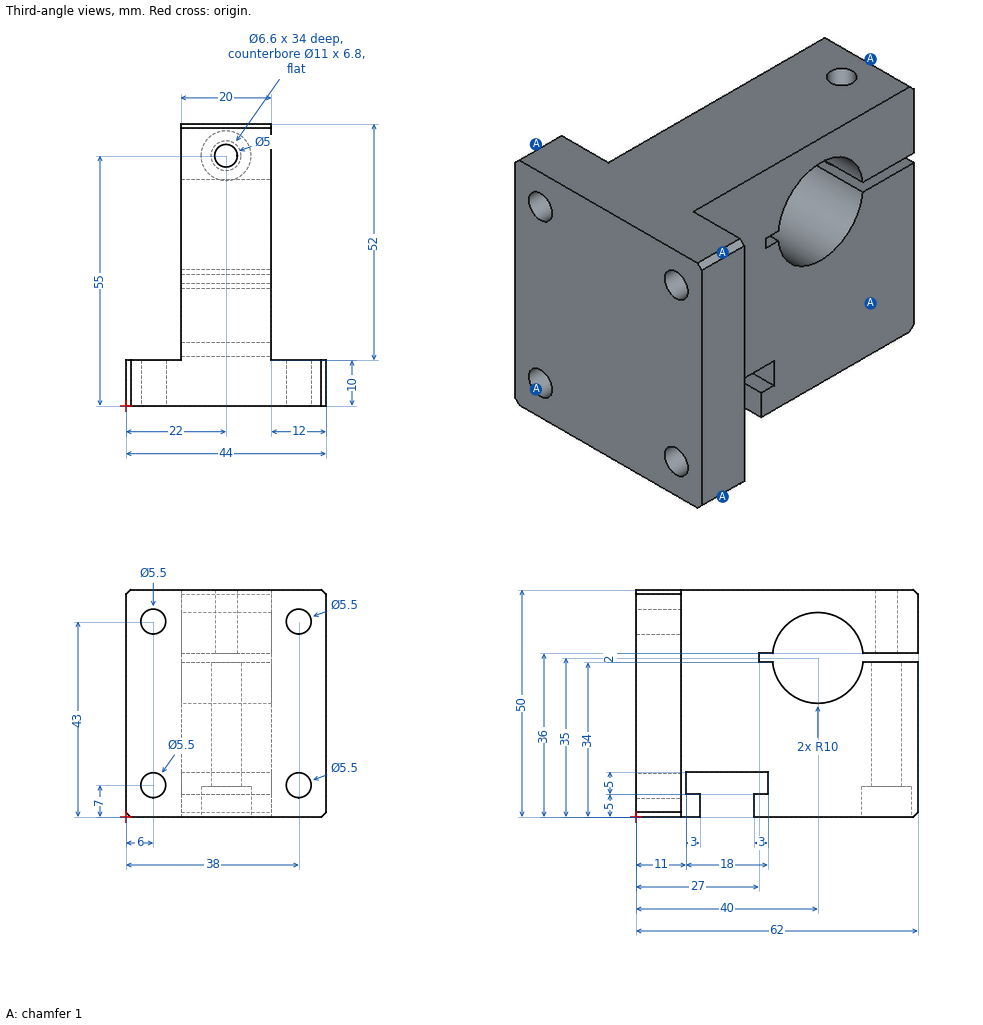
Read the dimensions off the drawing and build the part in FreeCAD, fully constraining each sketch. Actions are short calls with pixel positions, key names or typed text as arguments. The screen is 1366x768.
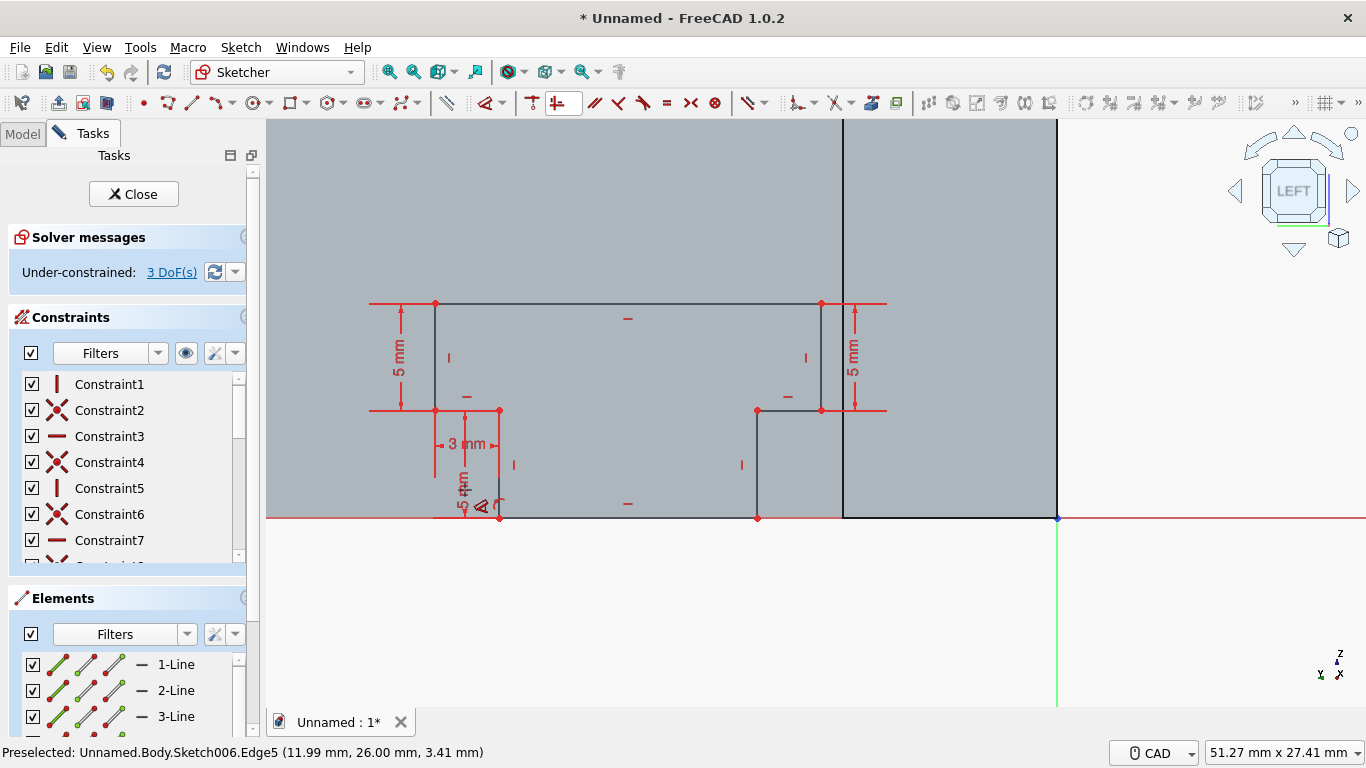
click(776, 411)
click(789, 445)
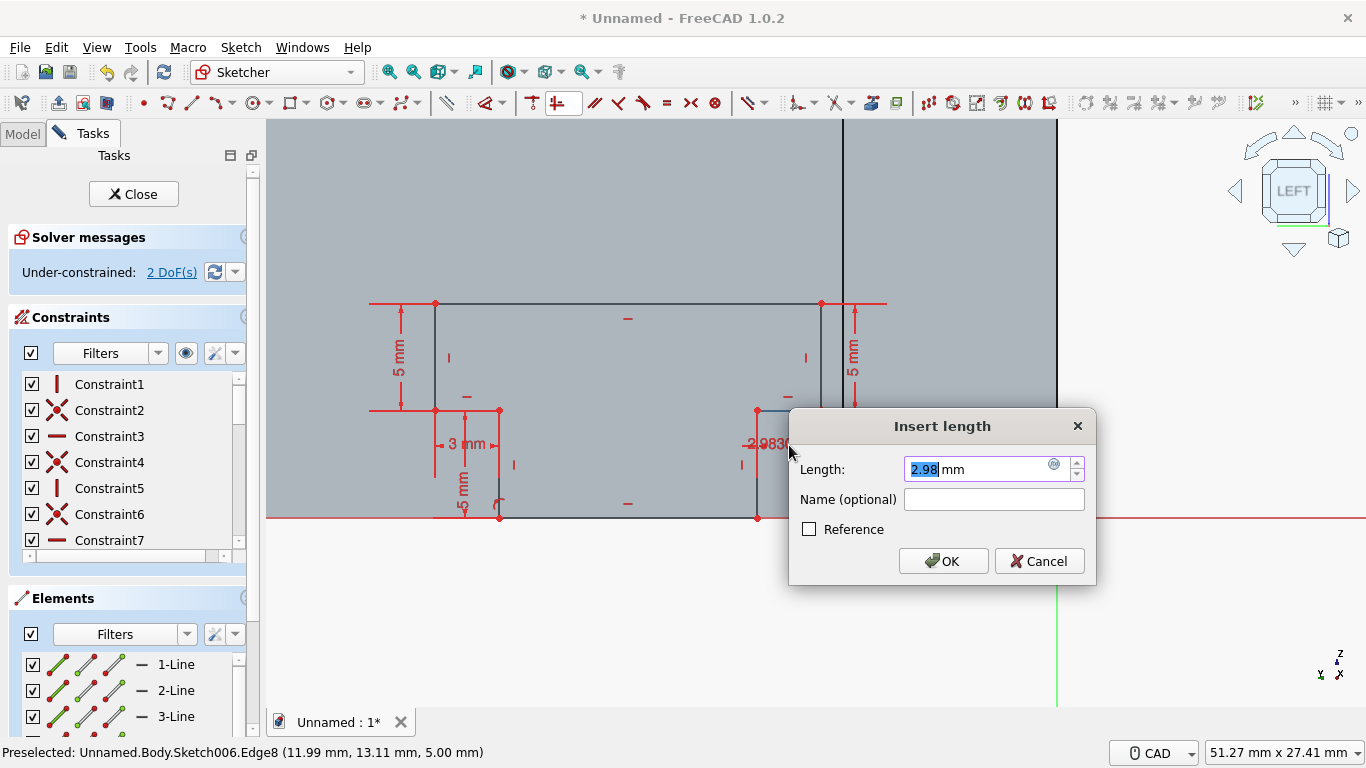
text(3)
key(Return)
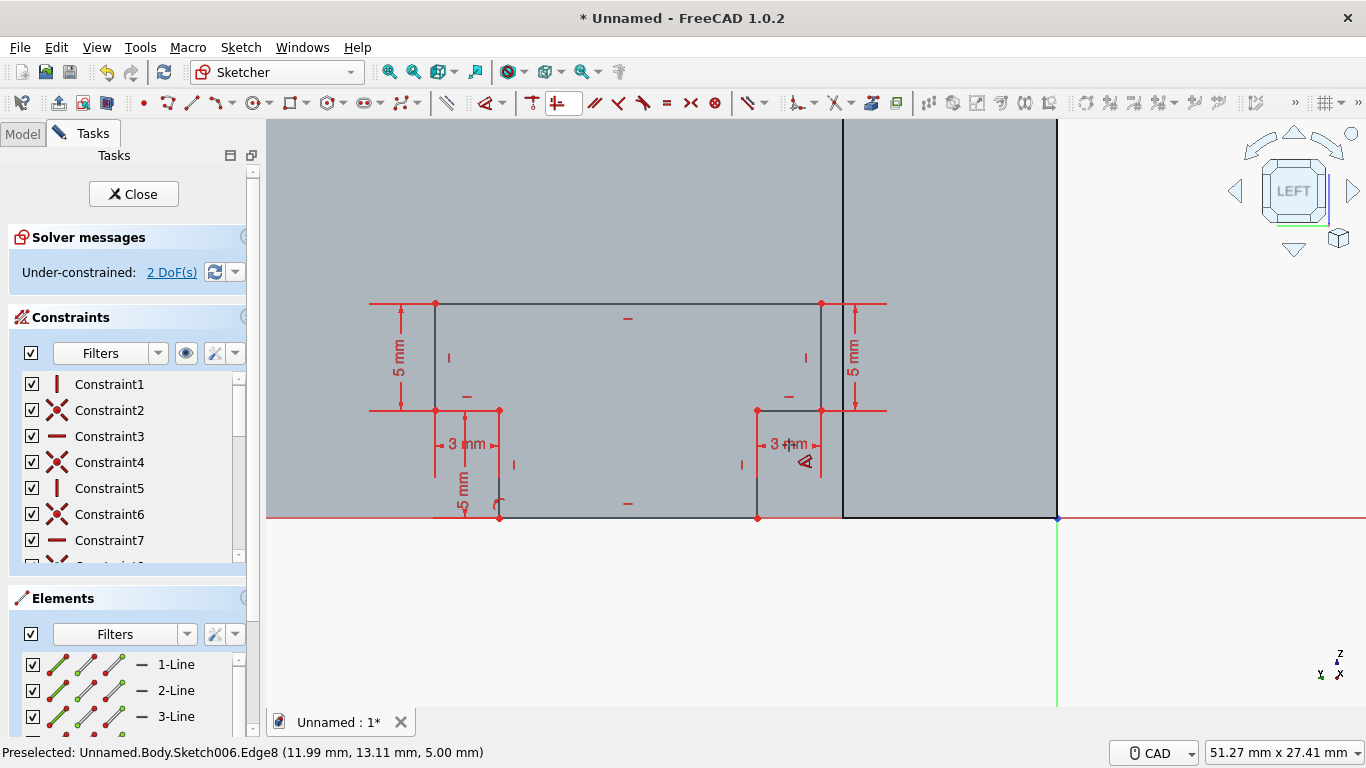
click(705, 304)
click(628, 270)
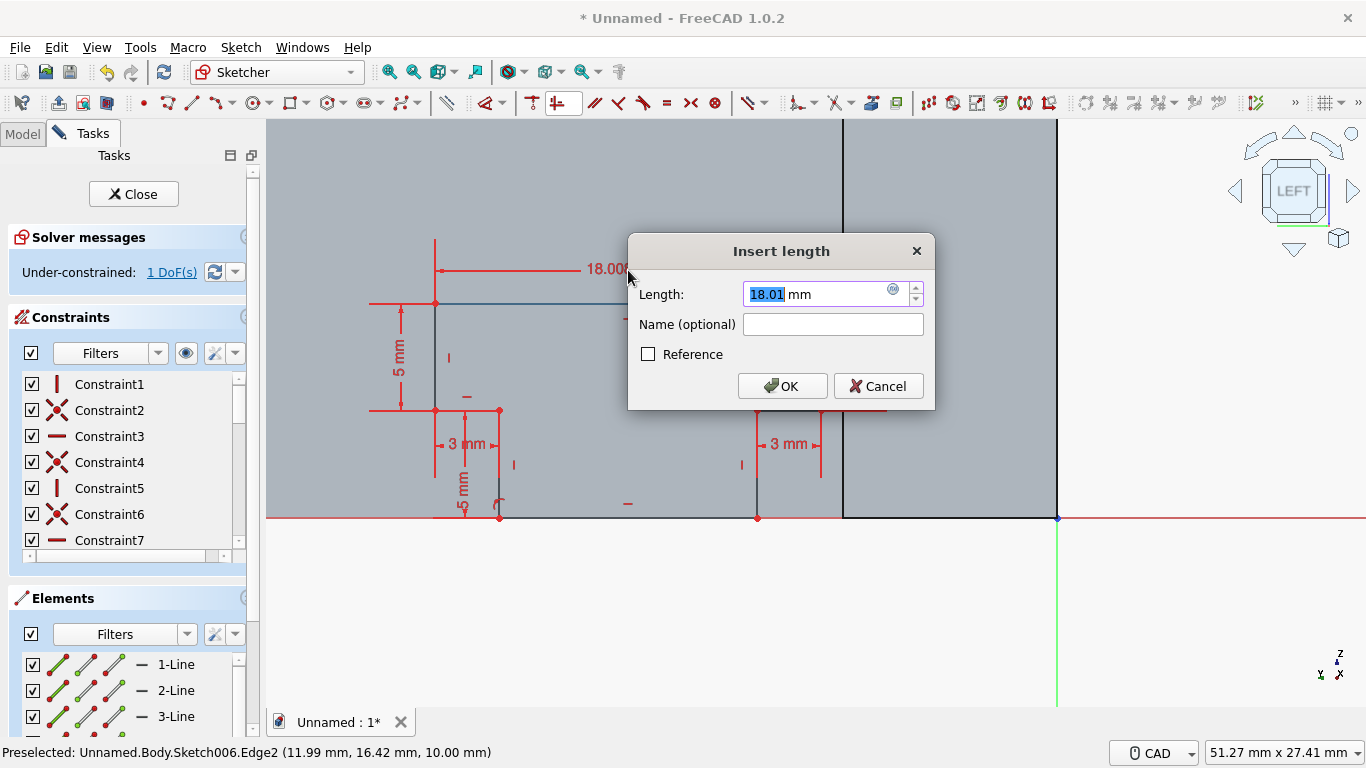
text(18)
key(Return)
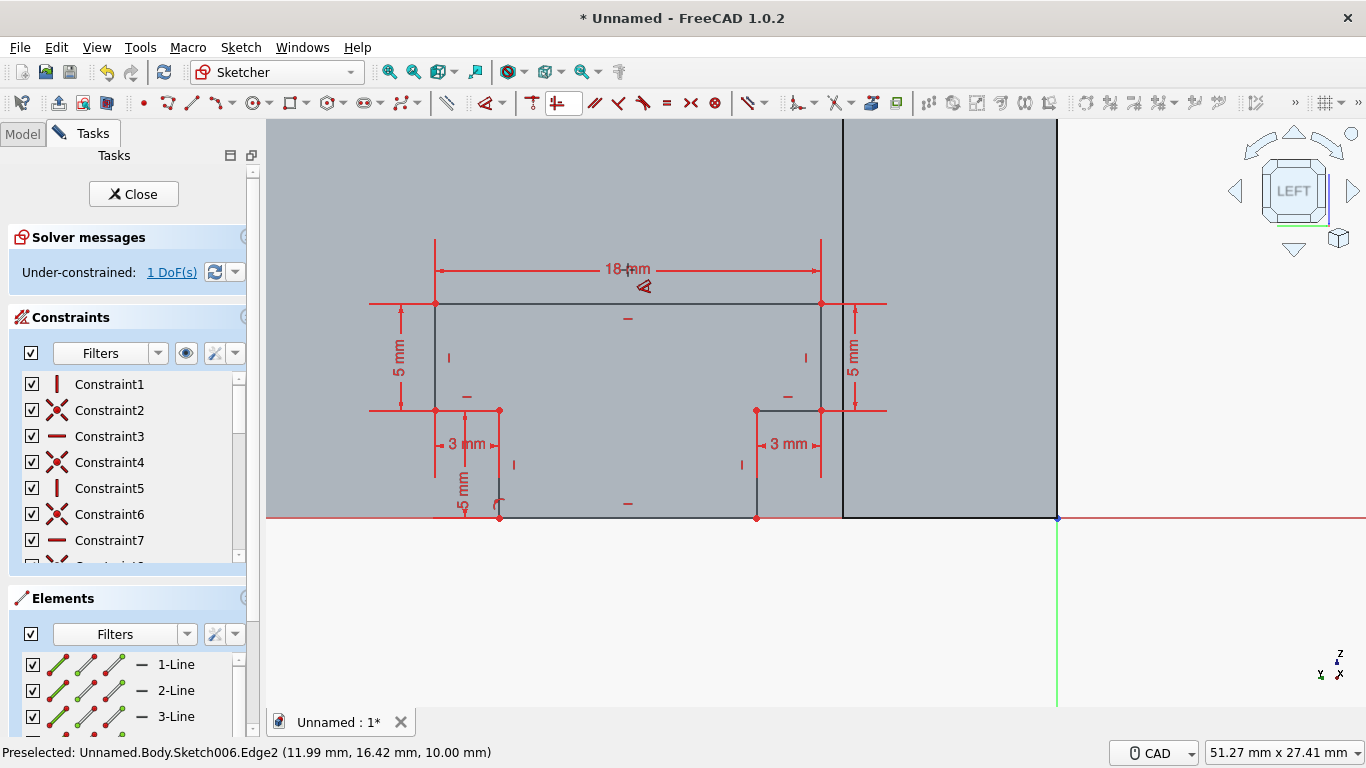
click(821, 411)
click(939, 552)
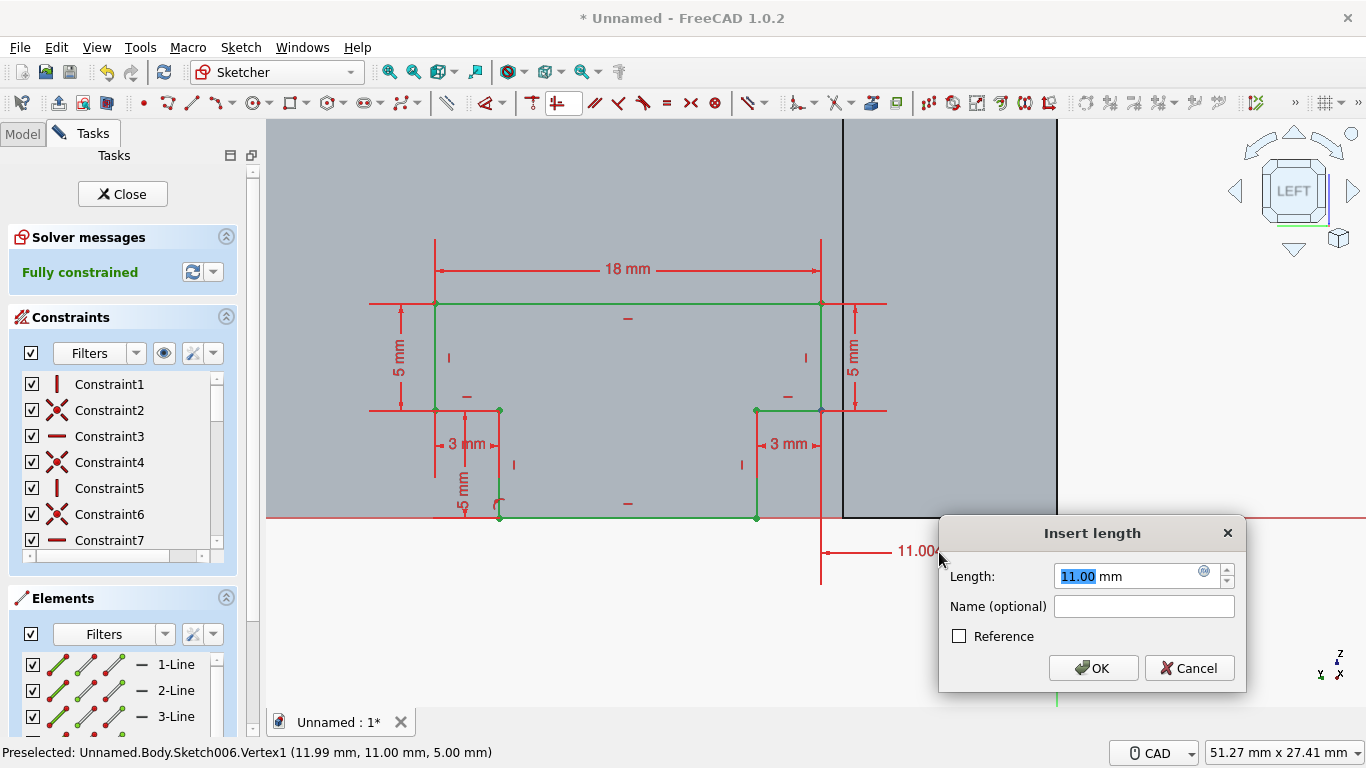
text(11)
key(Return)
key(Escape)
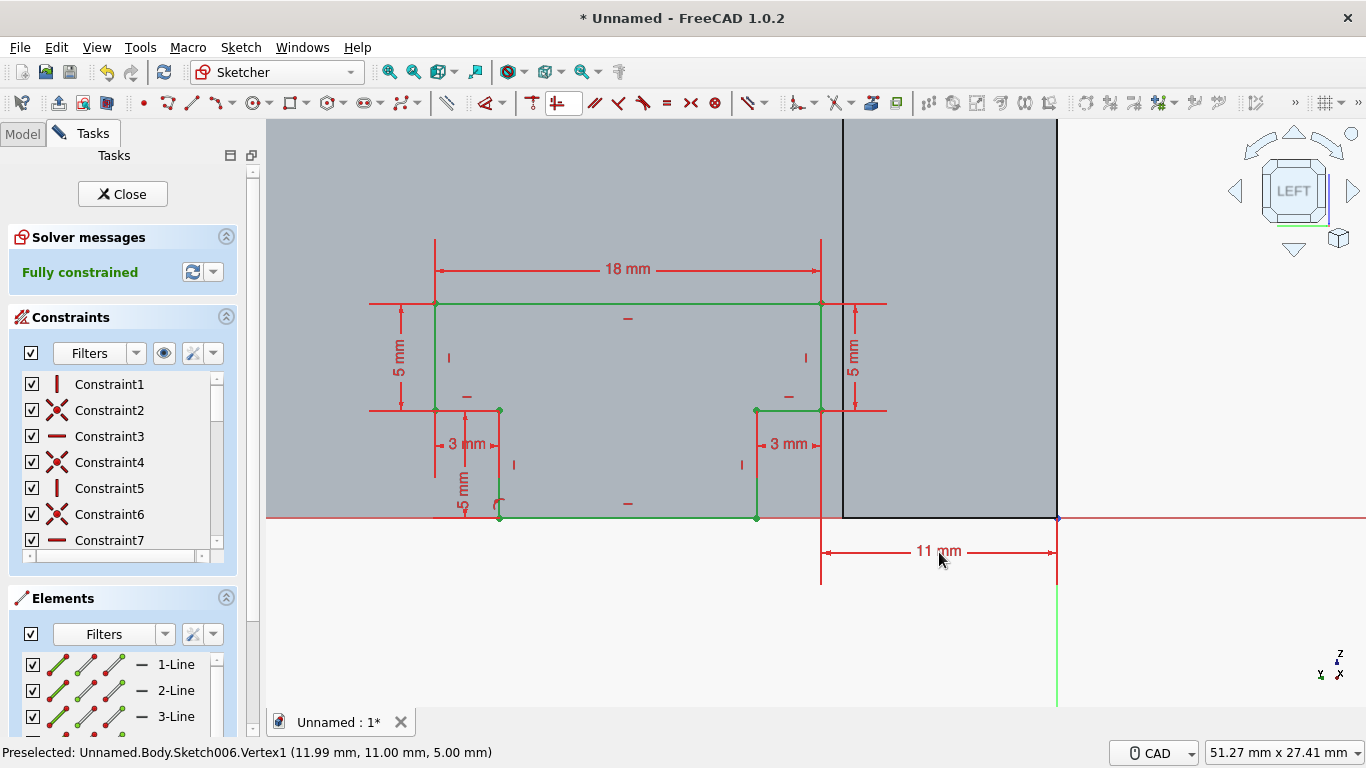
click(123, 194)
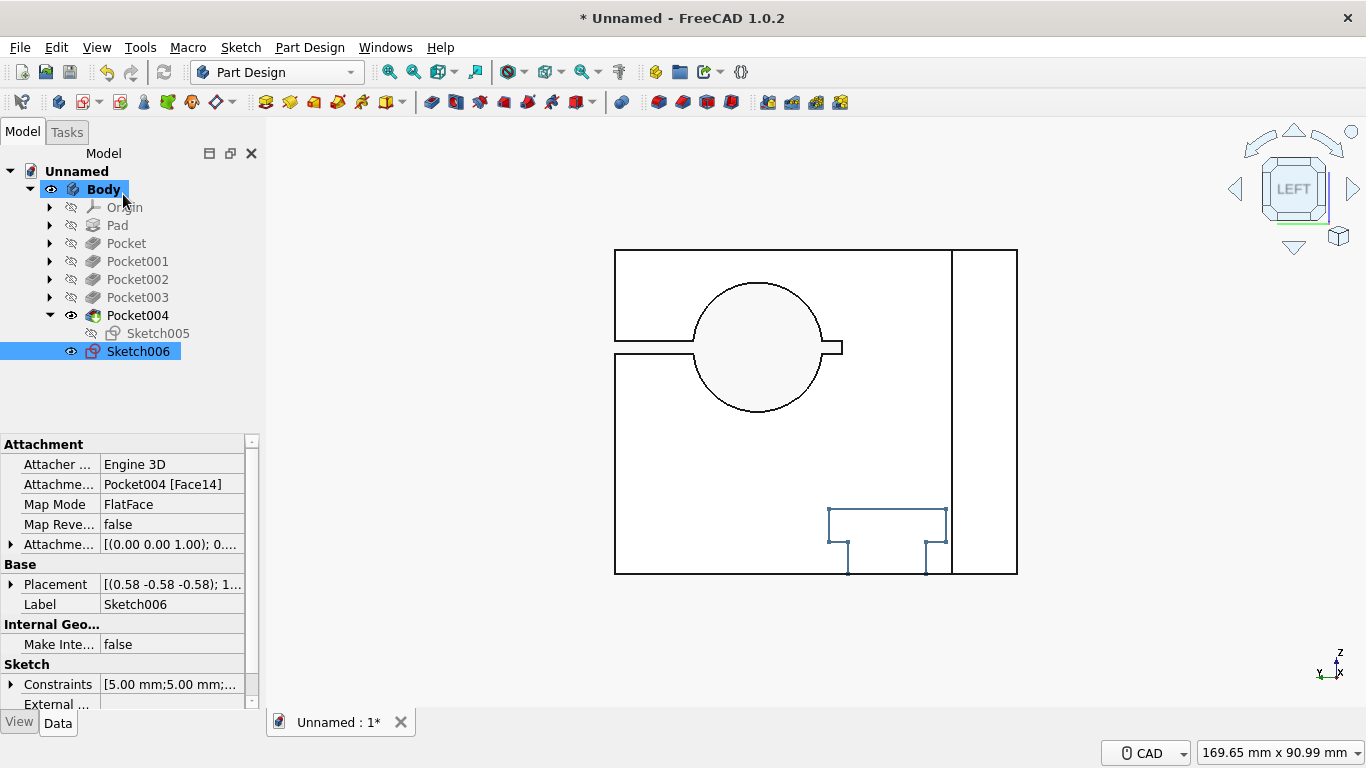
click(432, 102)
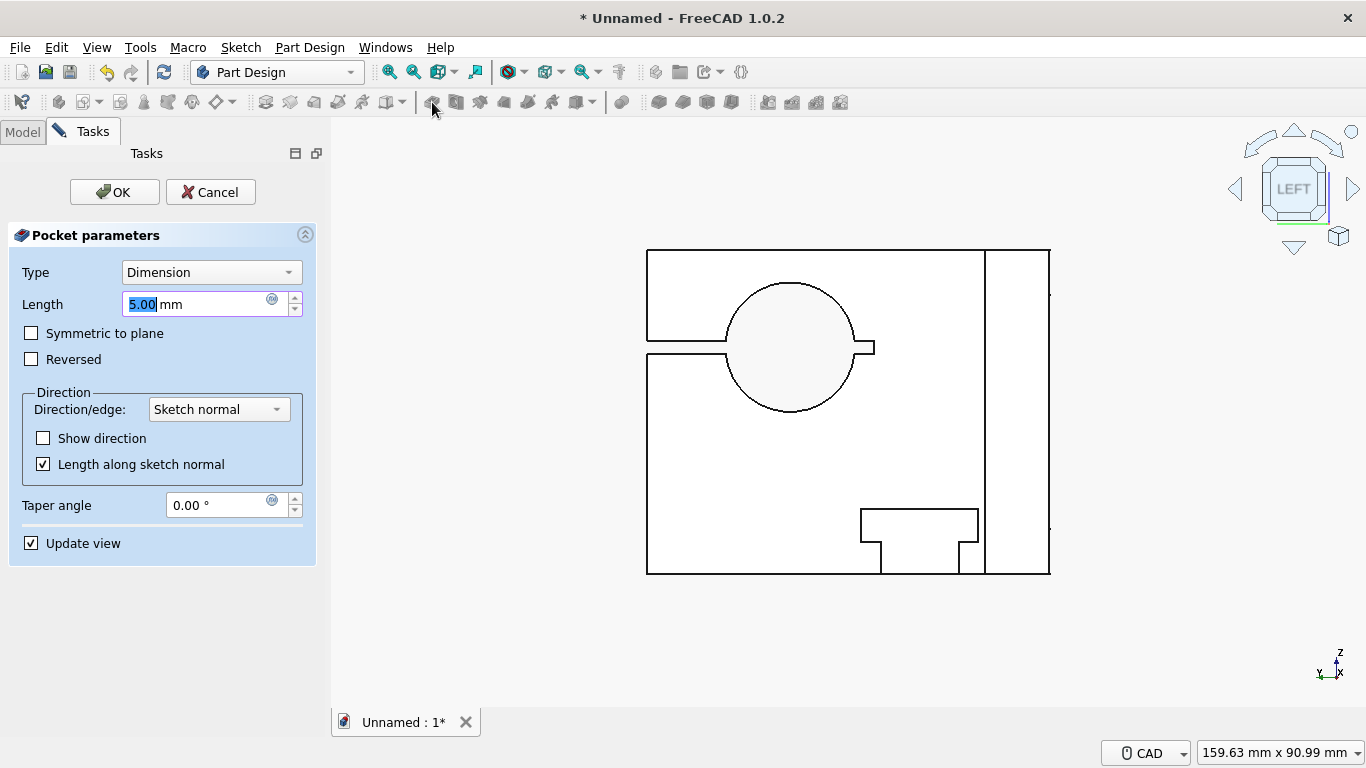
click(212, 272)